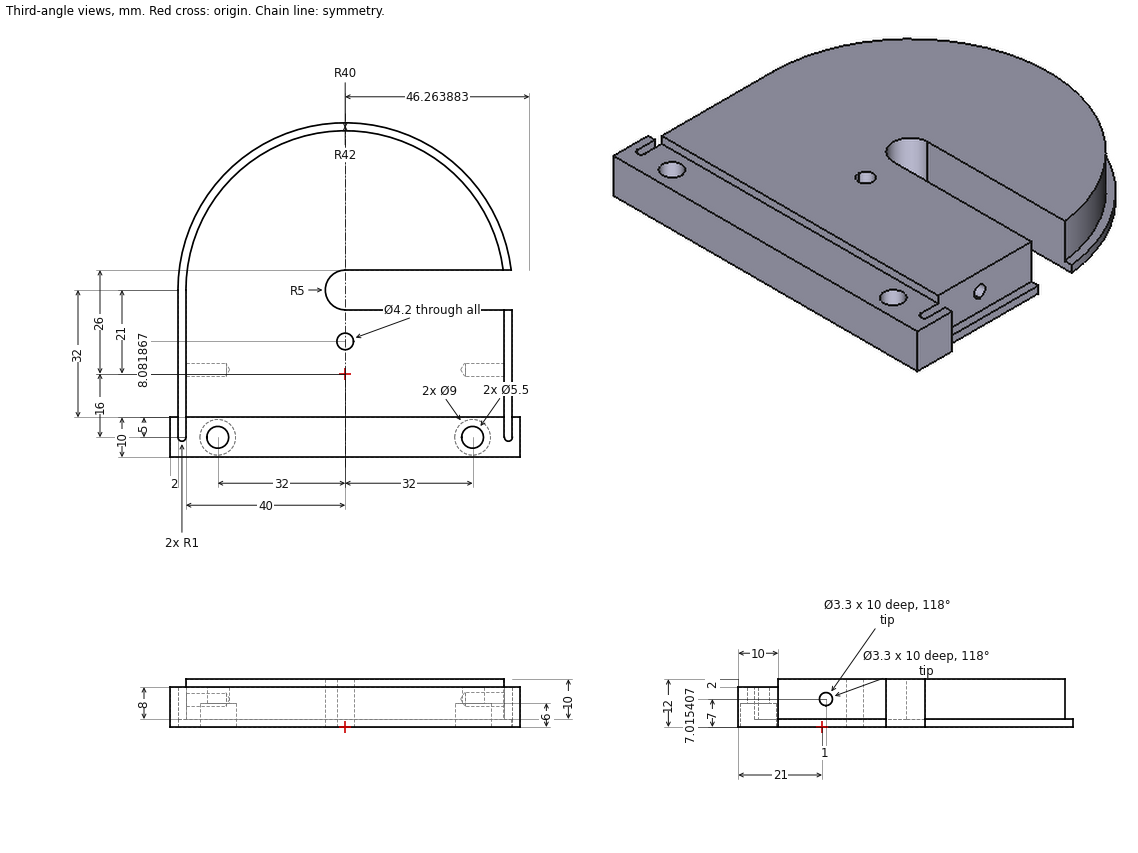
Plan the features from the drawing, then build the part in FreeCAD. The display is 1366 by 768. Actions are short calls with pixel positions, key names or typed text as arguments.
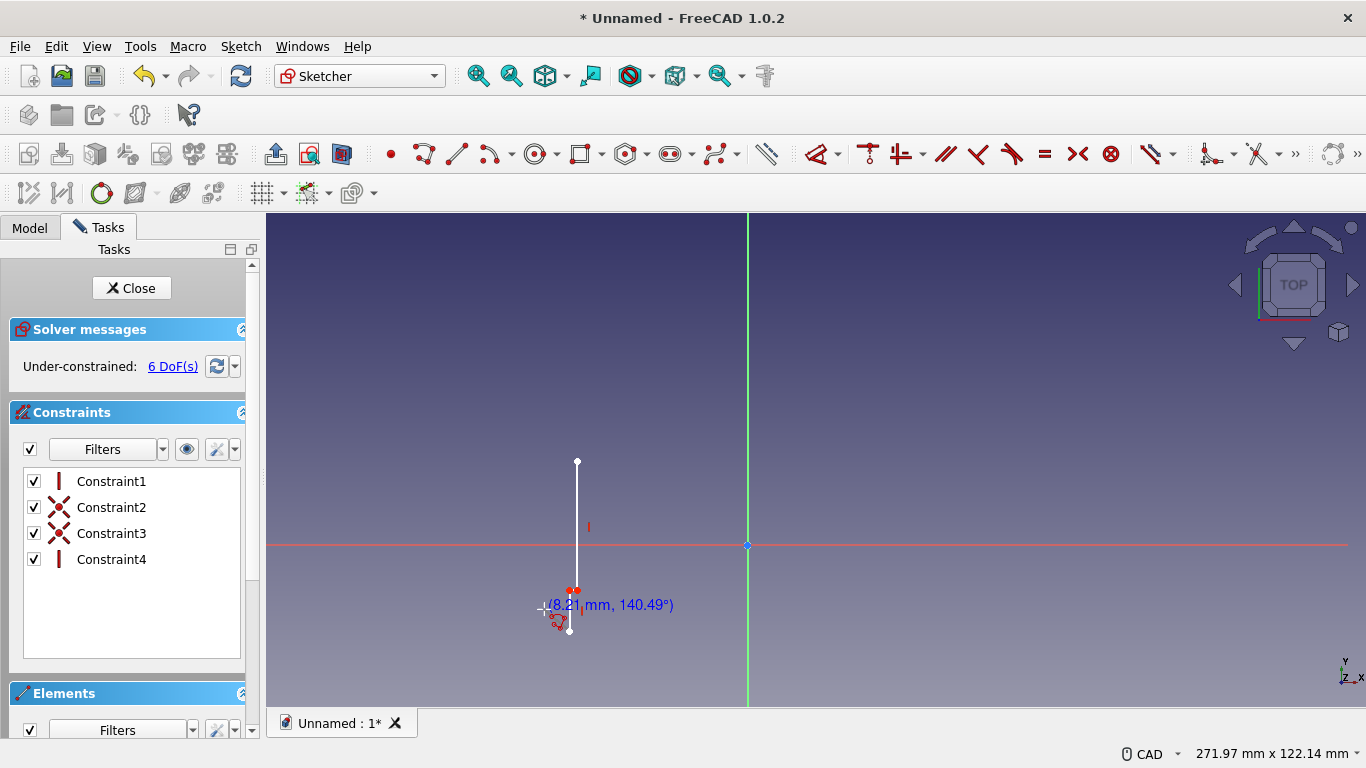
click(926, 631)
click(926, 590)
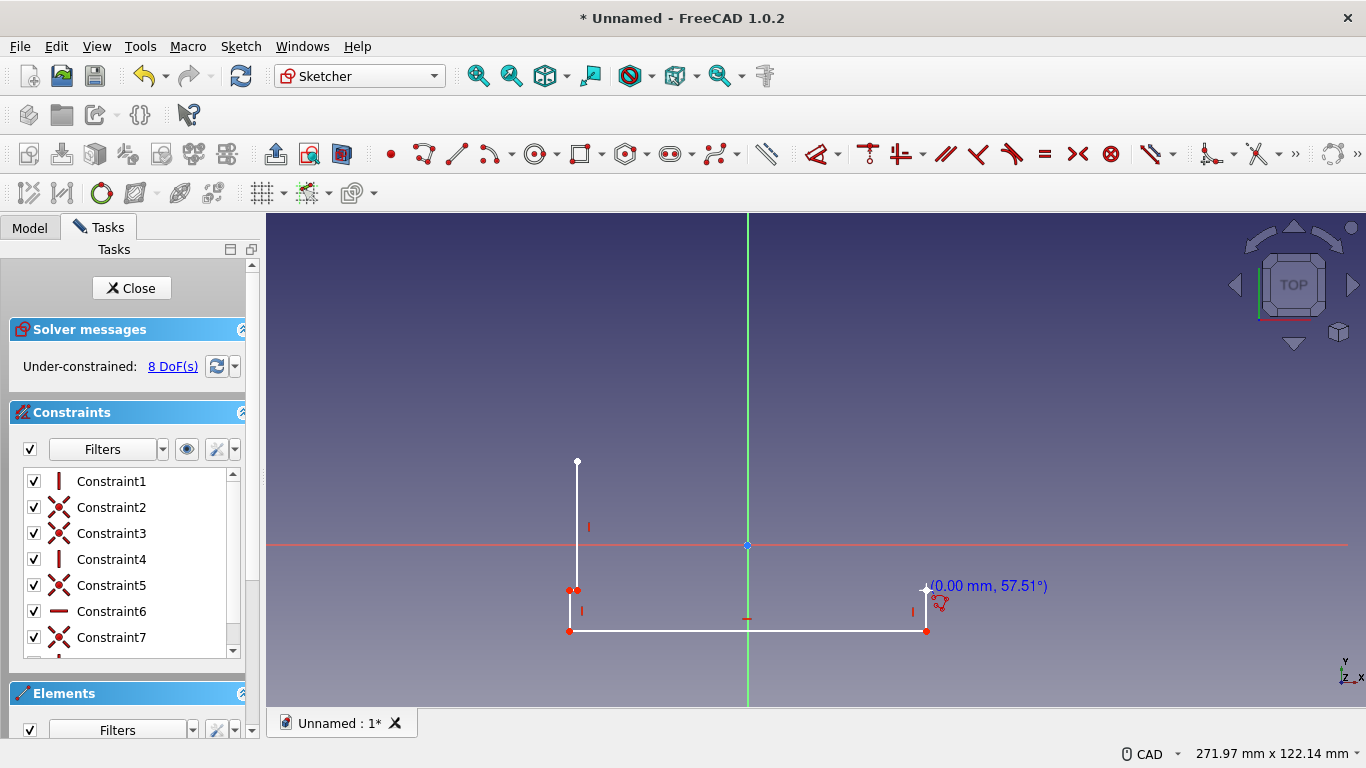
scroll(918, 590, up, 4)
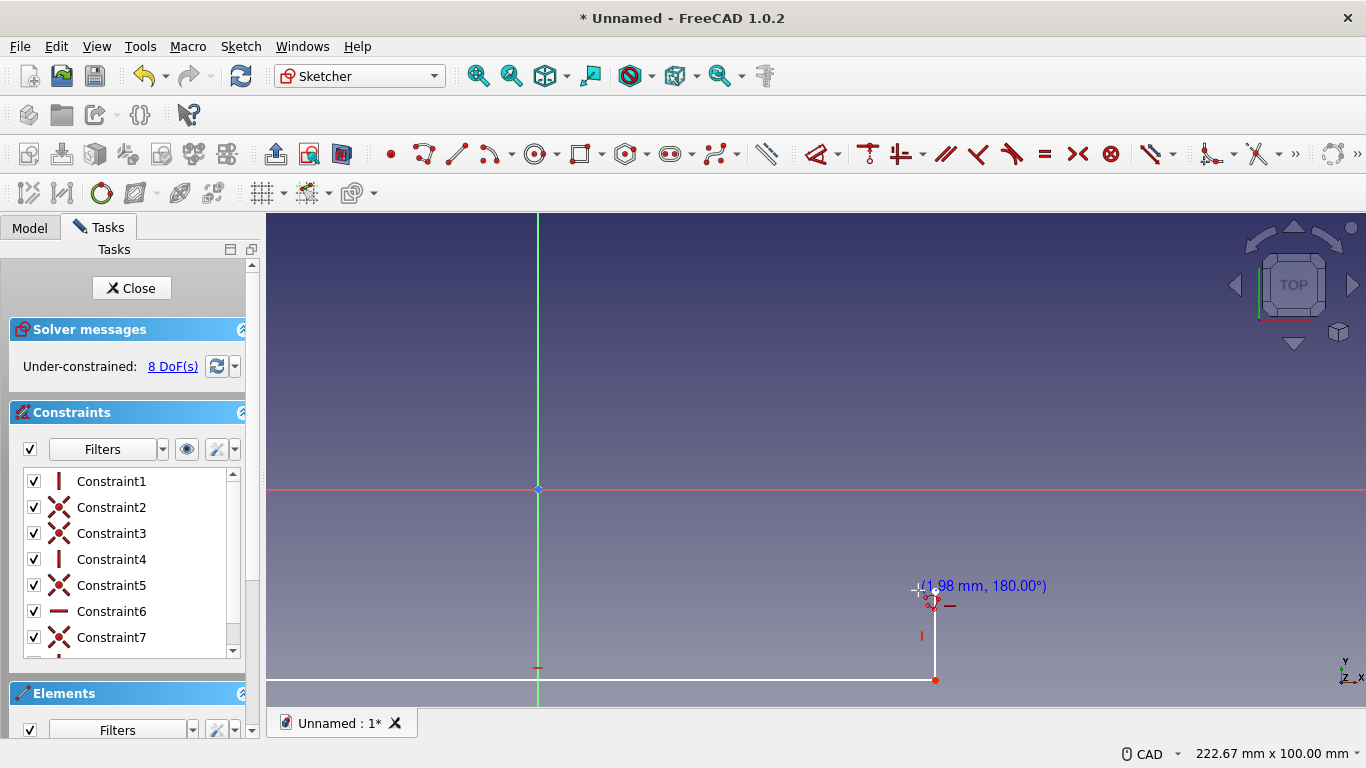
click(916, 589)
click(916, 301)
right_click(916, 301)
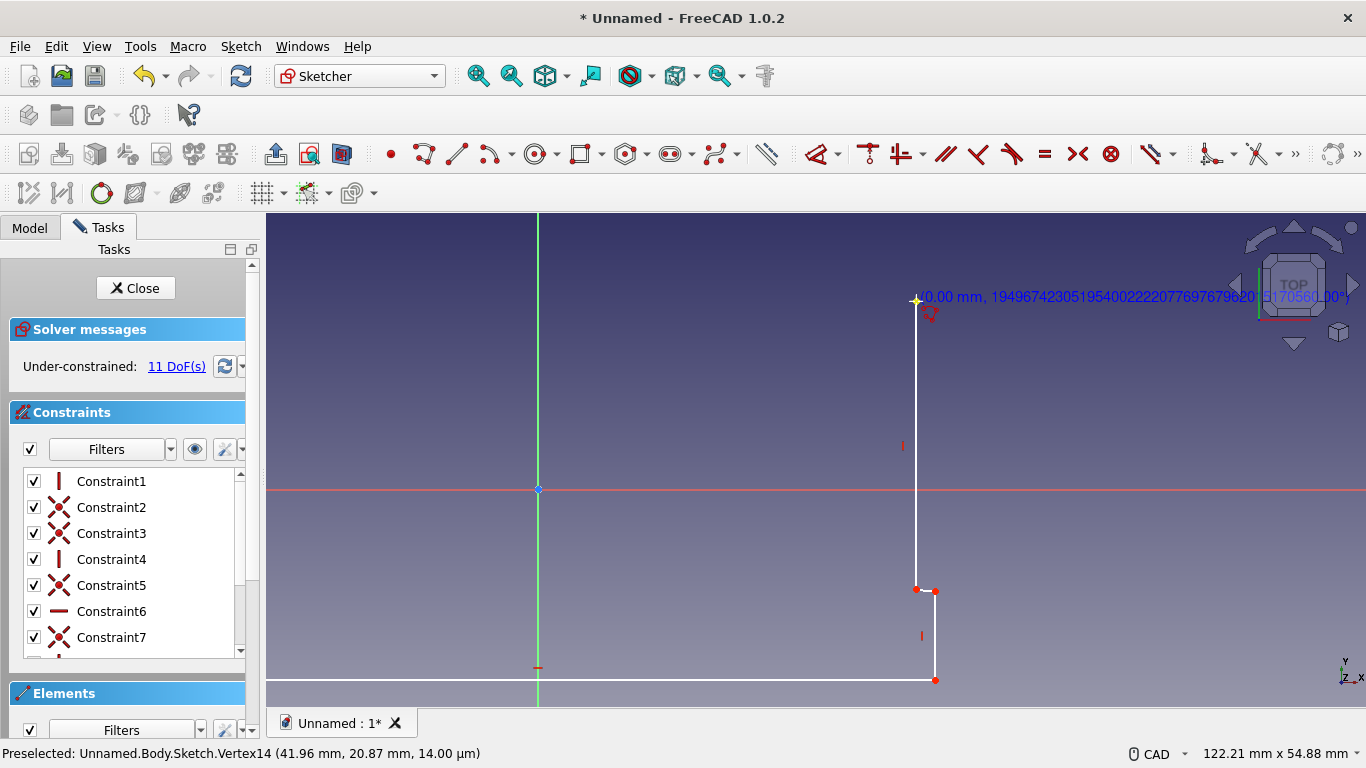
click(512, 154)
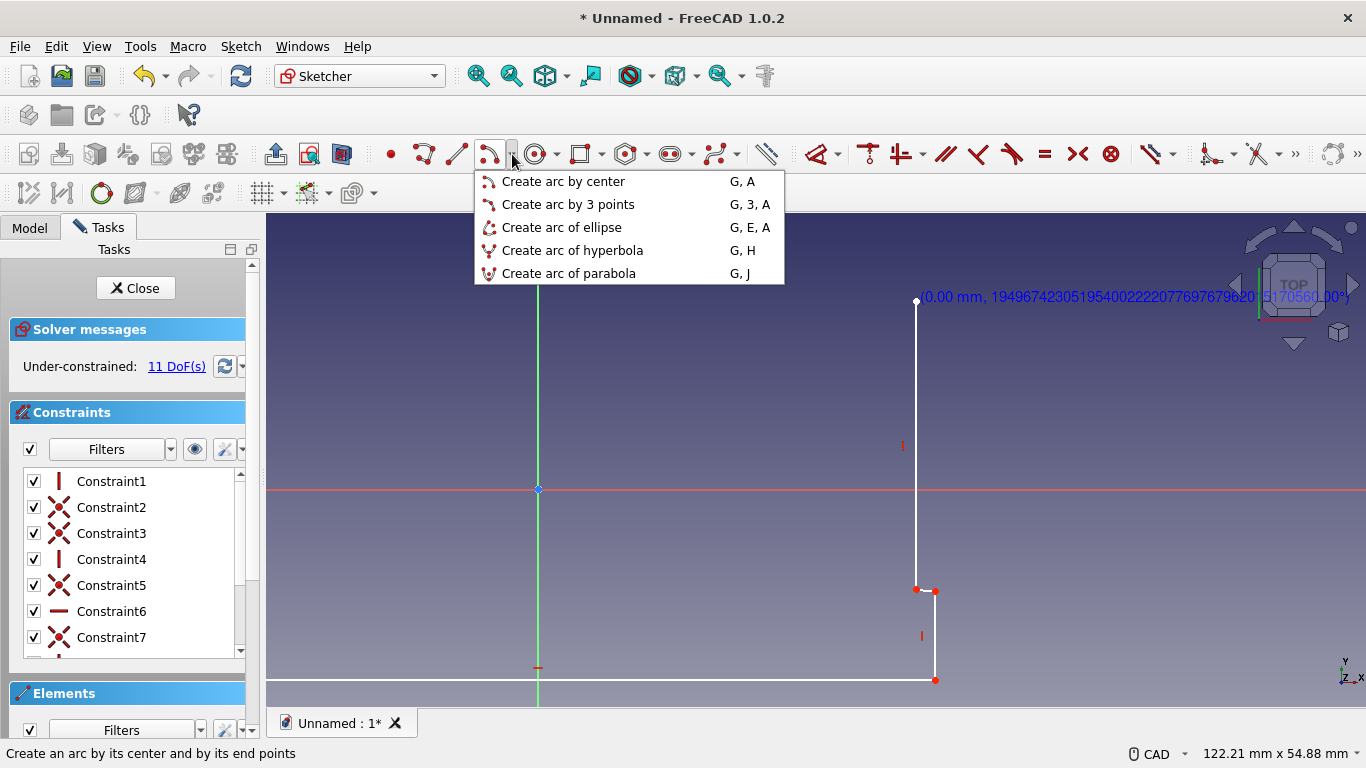
click(630, 204)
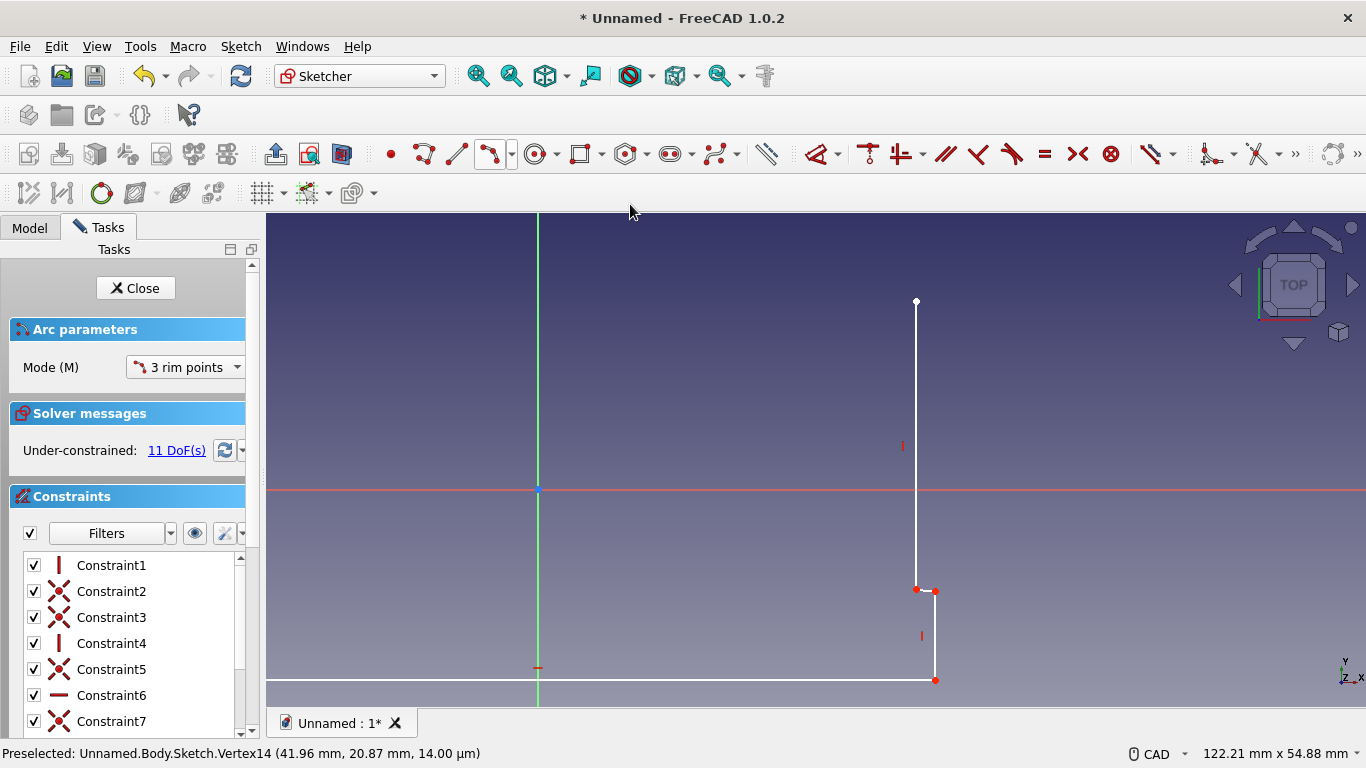
click(916, 302)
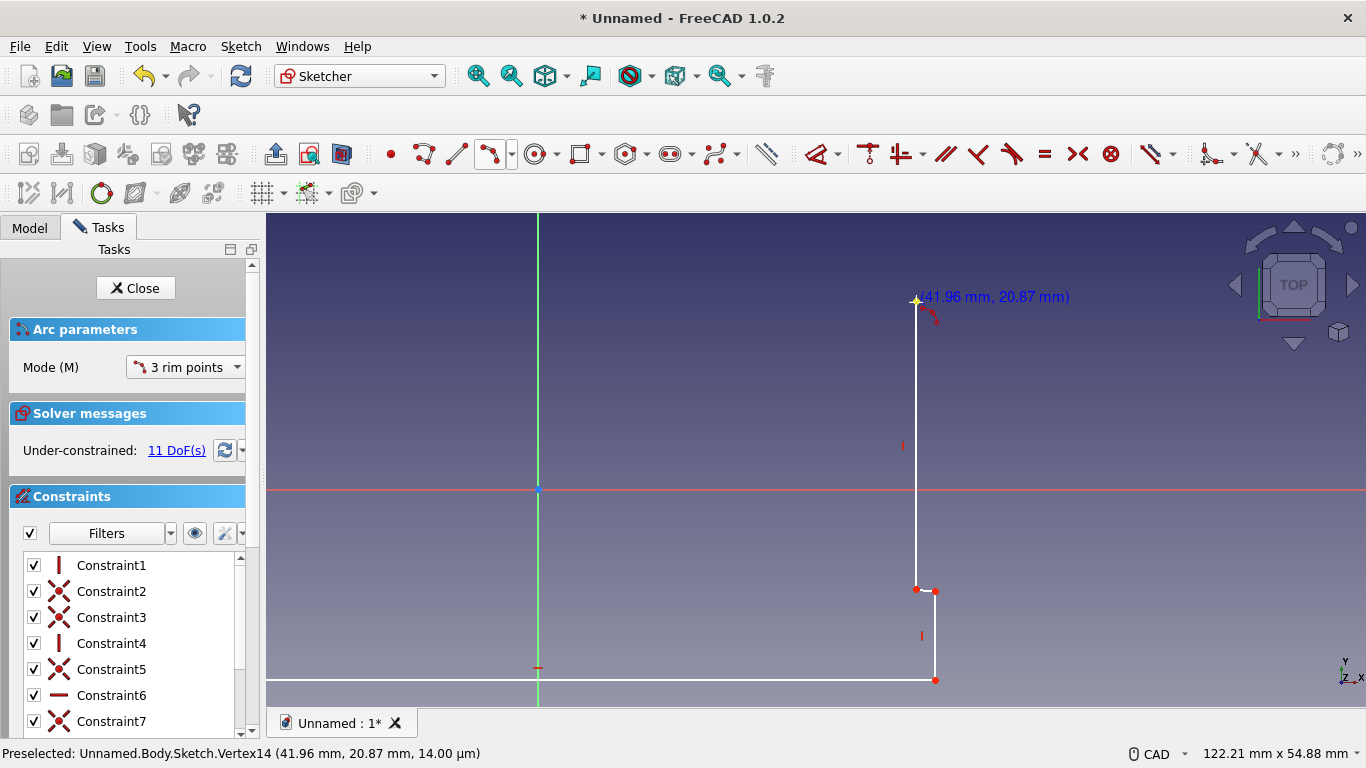
scroll(918, 590, down, 4)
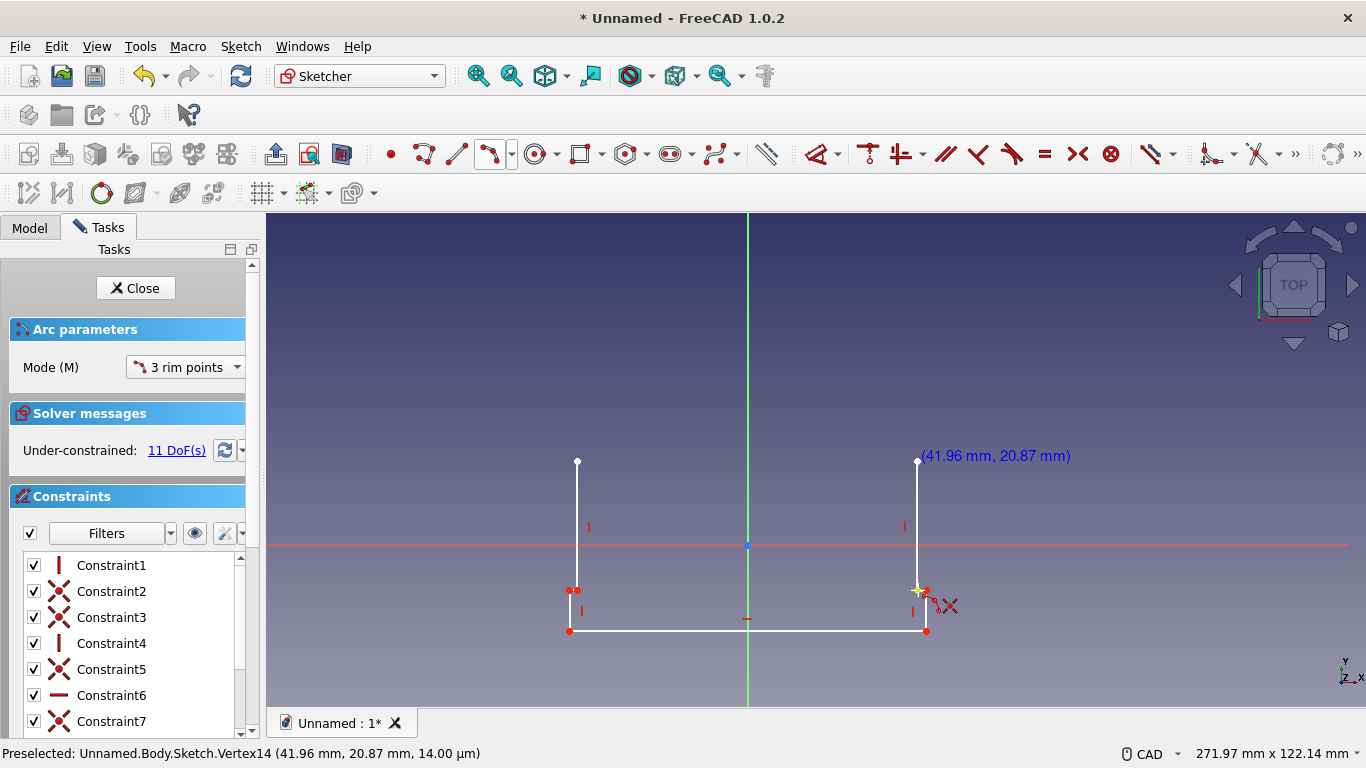
click(577, 461)
click(800, 299)
key(Escape)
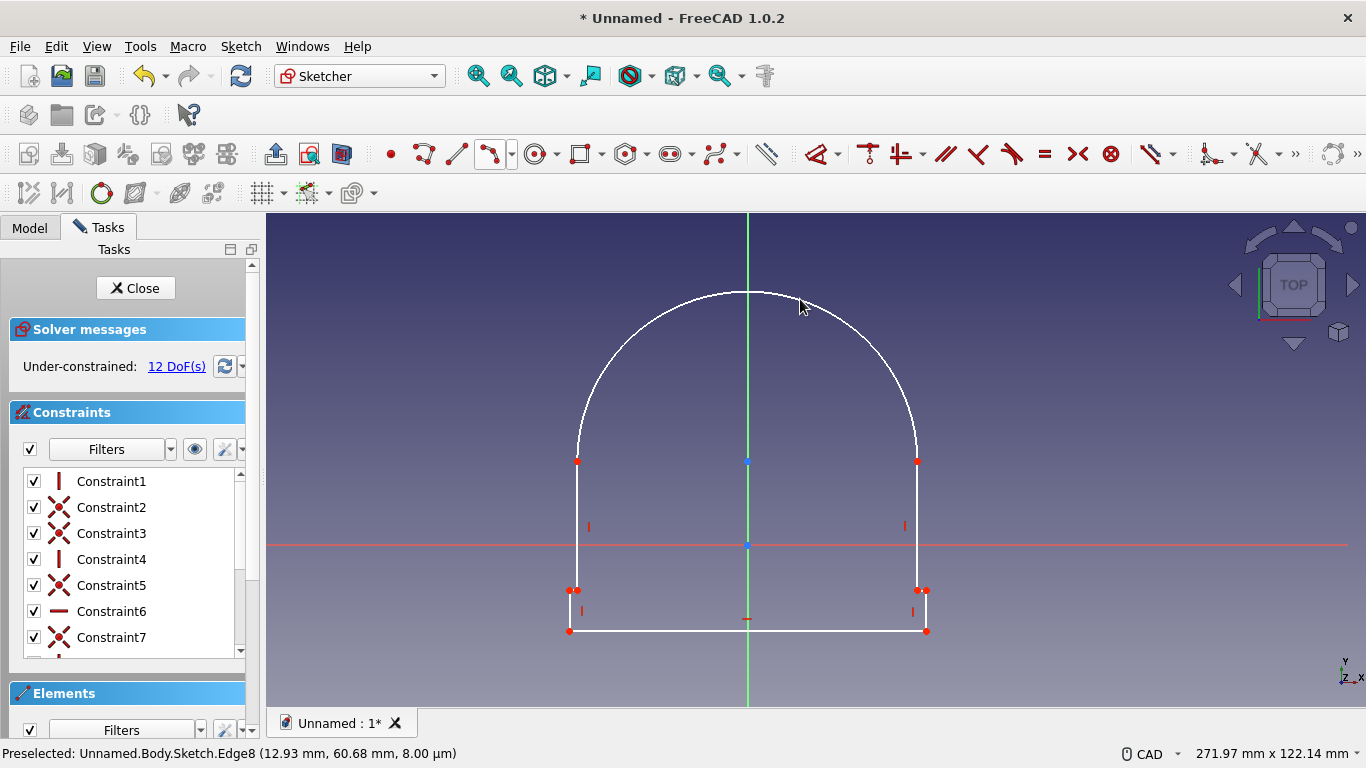
scroll(574, 590, up, 7)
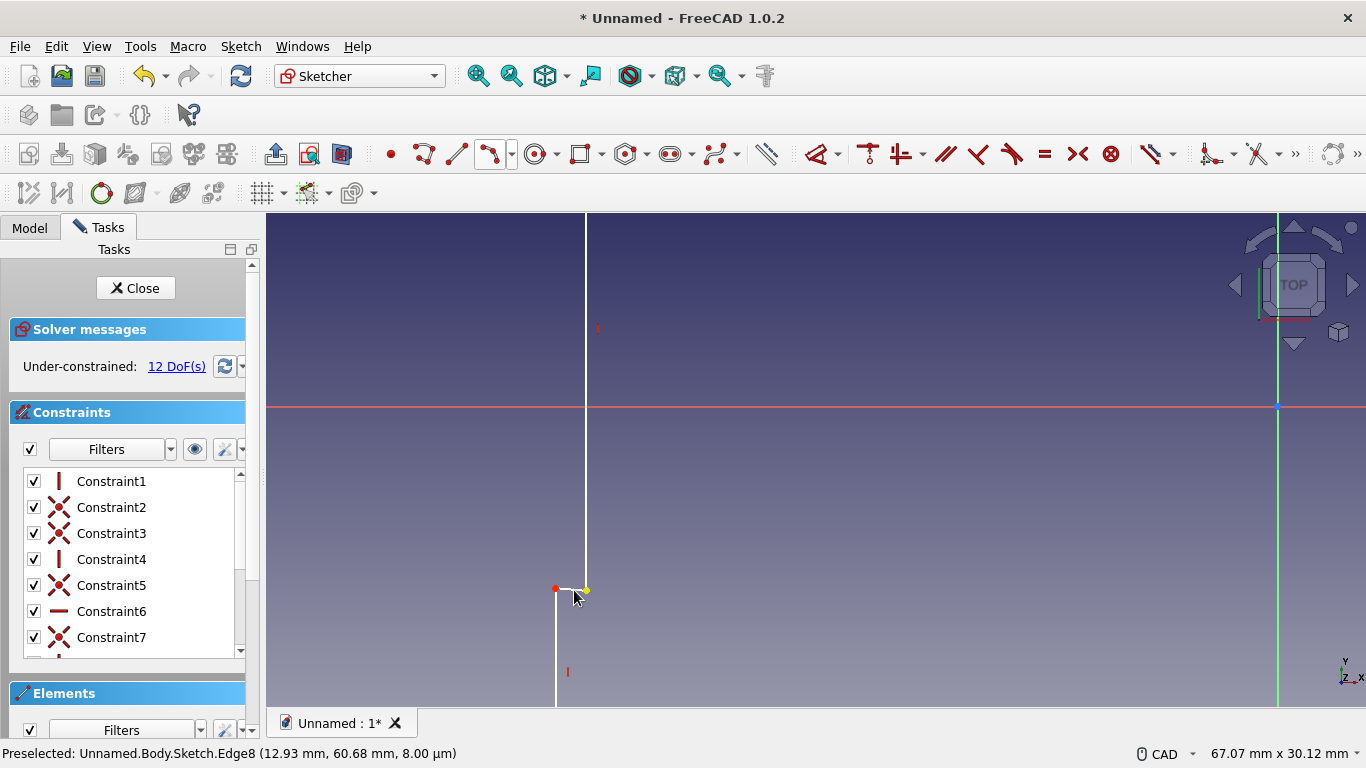
click(571, 590)